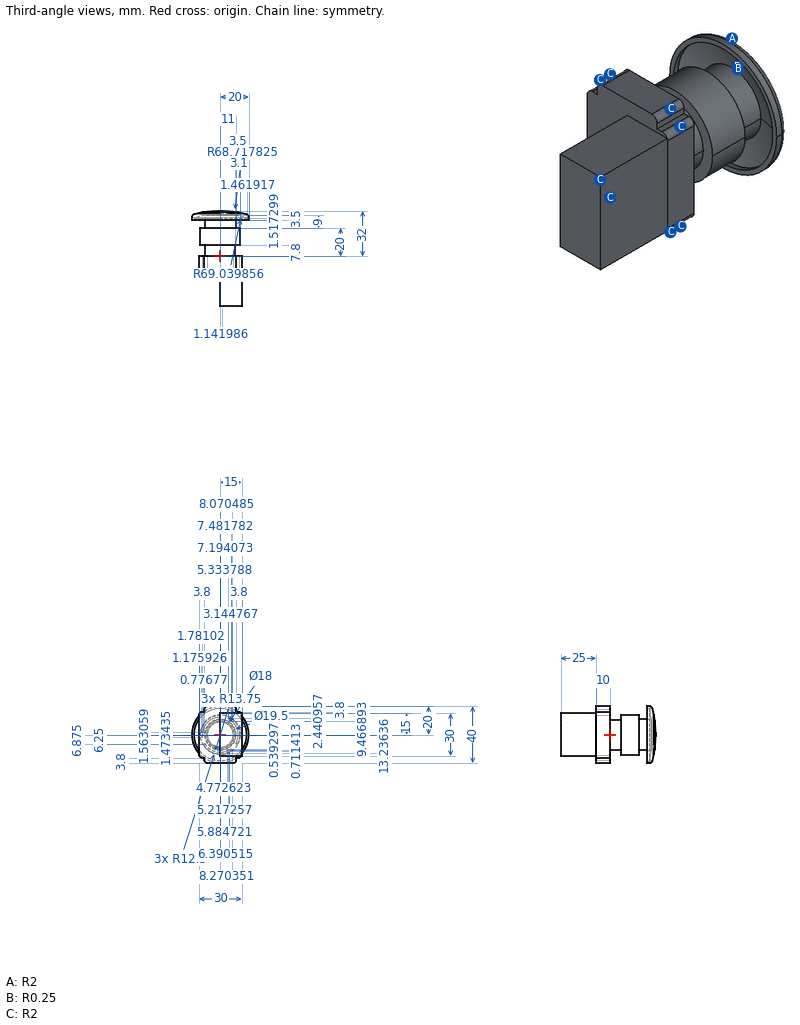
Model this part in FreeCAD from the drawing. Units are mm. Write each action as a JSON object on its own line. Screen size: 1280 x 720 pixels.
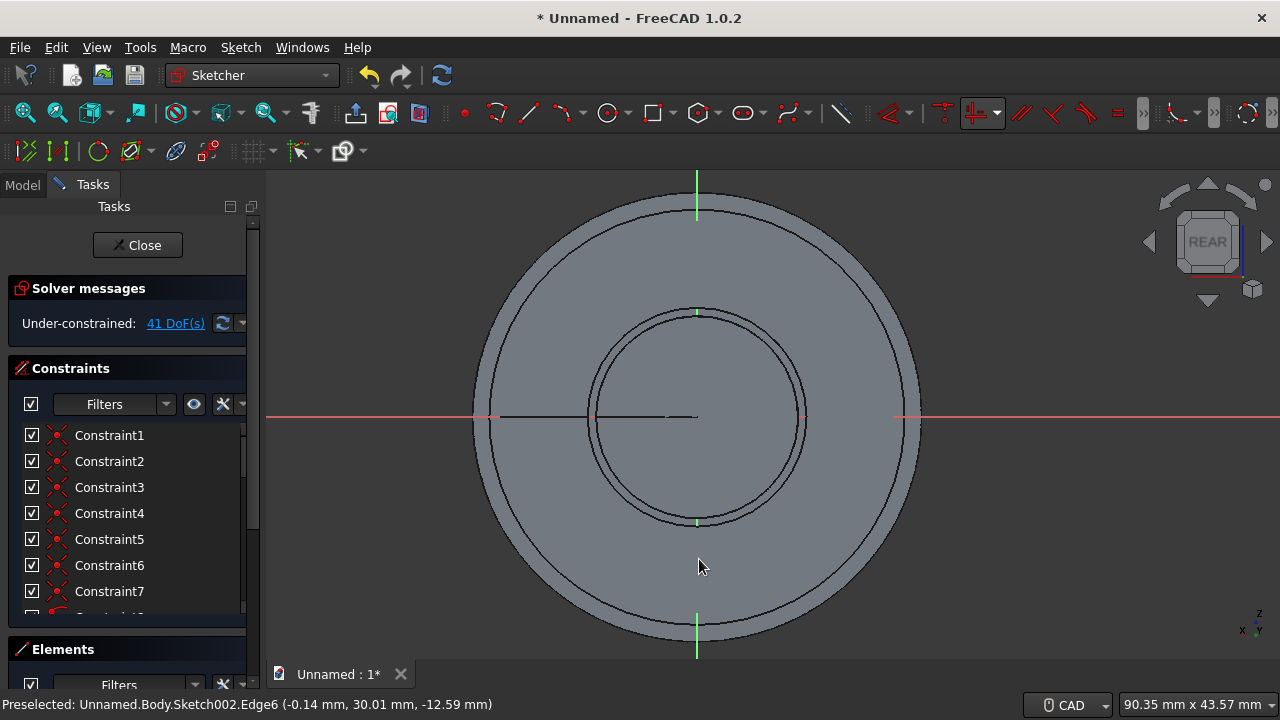
{"action": "left_click", "coordinate": [816, 344]}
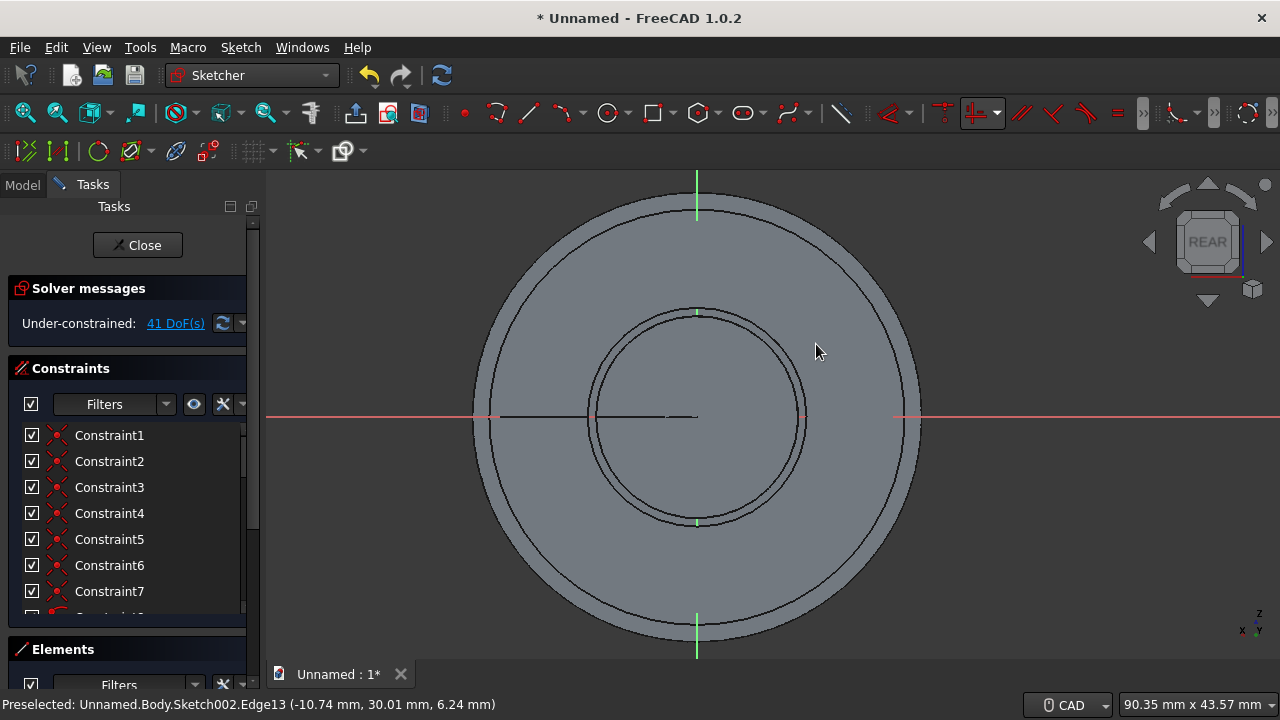
{"action": "left_click", "coordinate": [944, 114]}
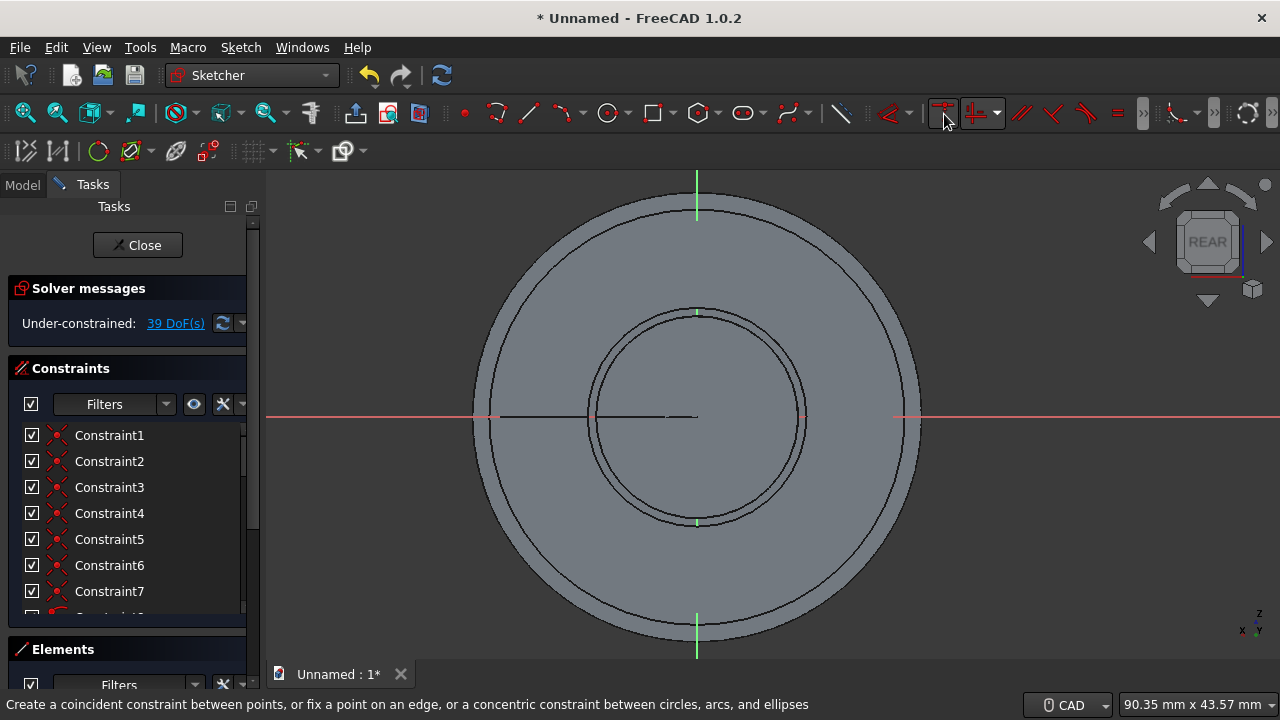
{"action": "left_click", "coordinate": [699, 558]}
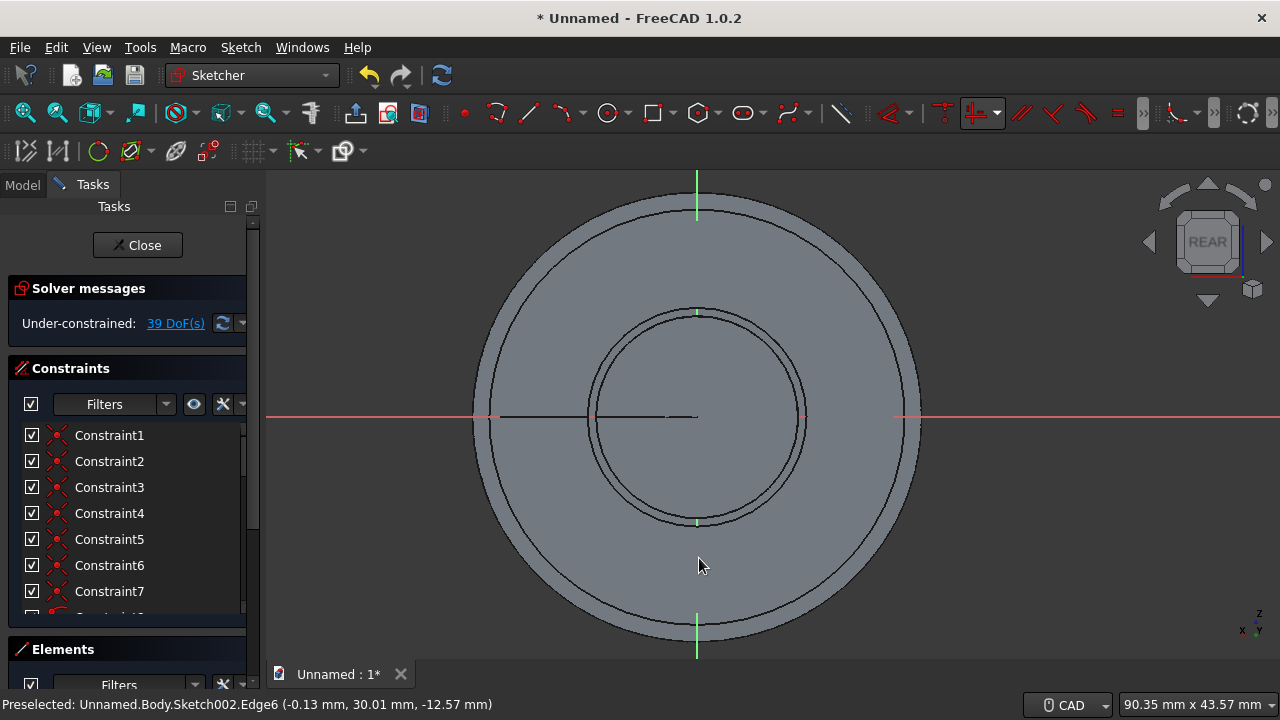
{"action": "left_click", "coordinate": [829, 337]}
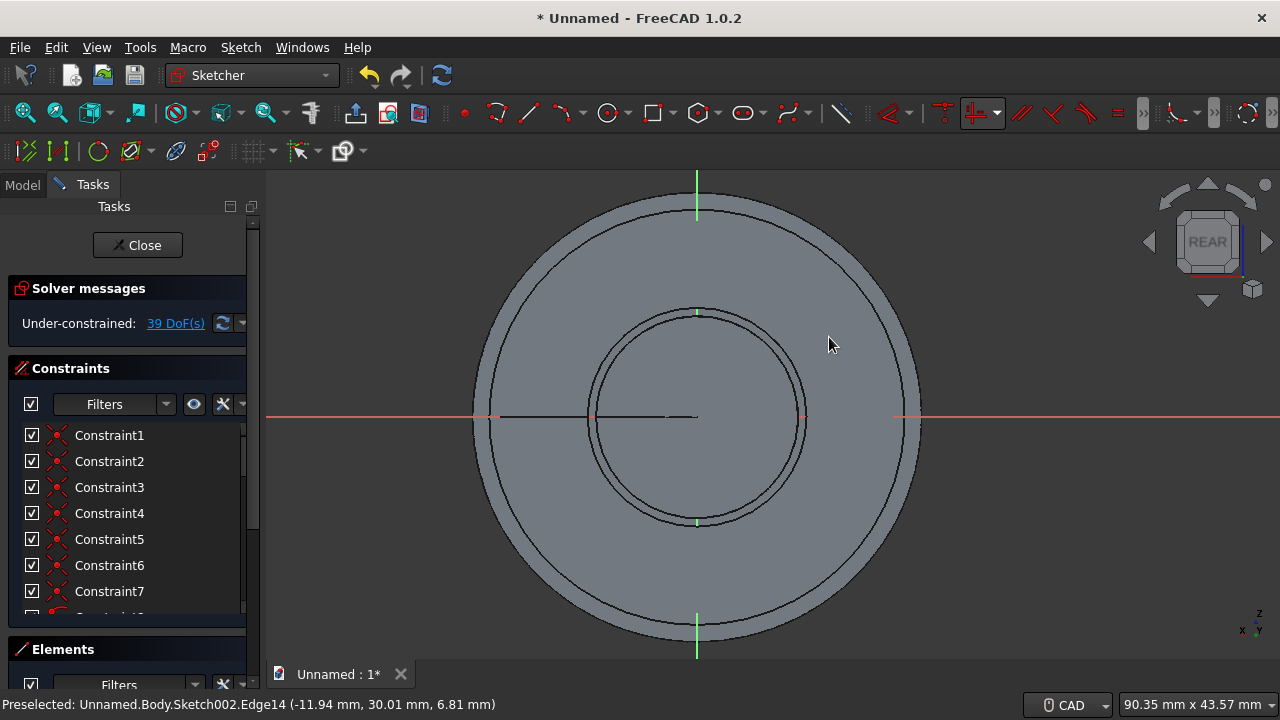
{"action": "left_click", "coordinate": [944, 114]}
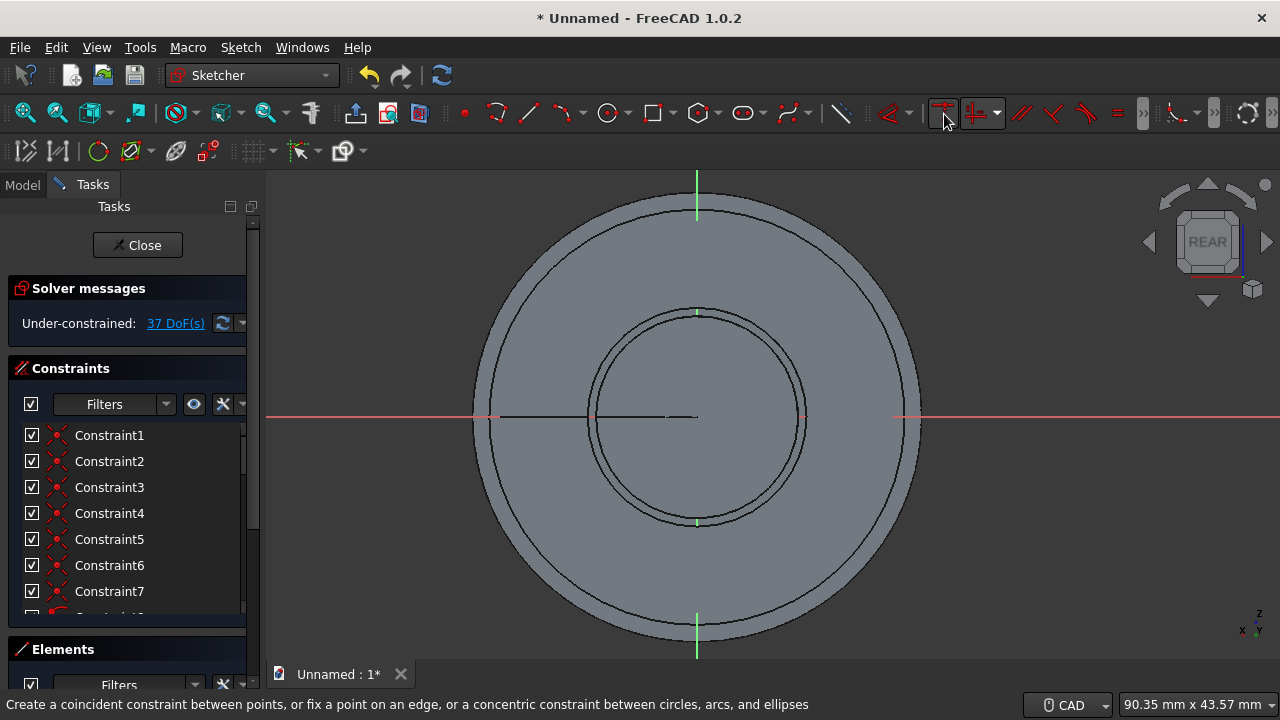
{"action": "left_click", "coordinate": [699, 558]}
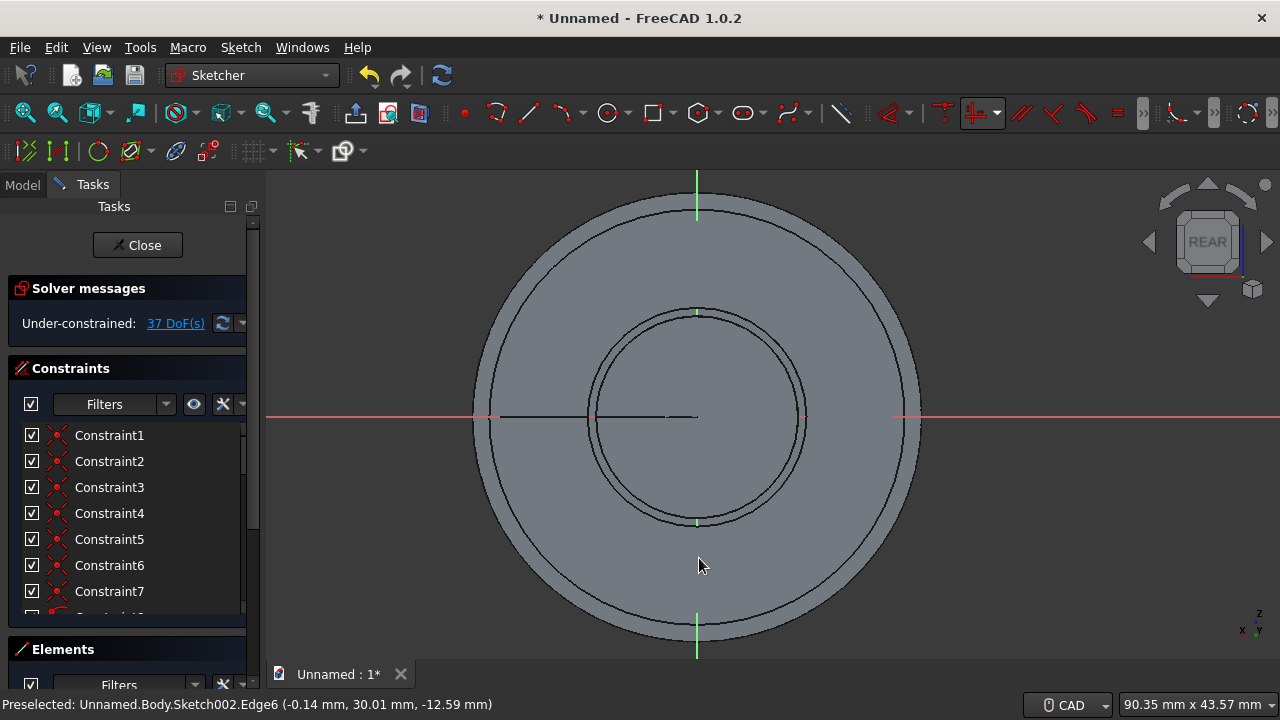
{"action": "left_click", "coordinate": [574, 352]}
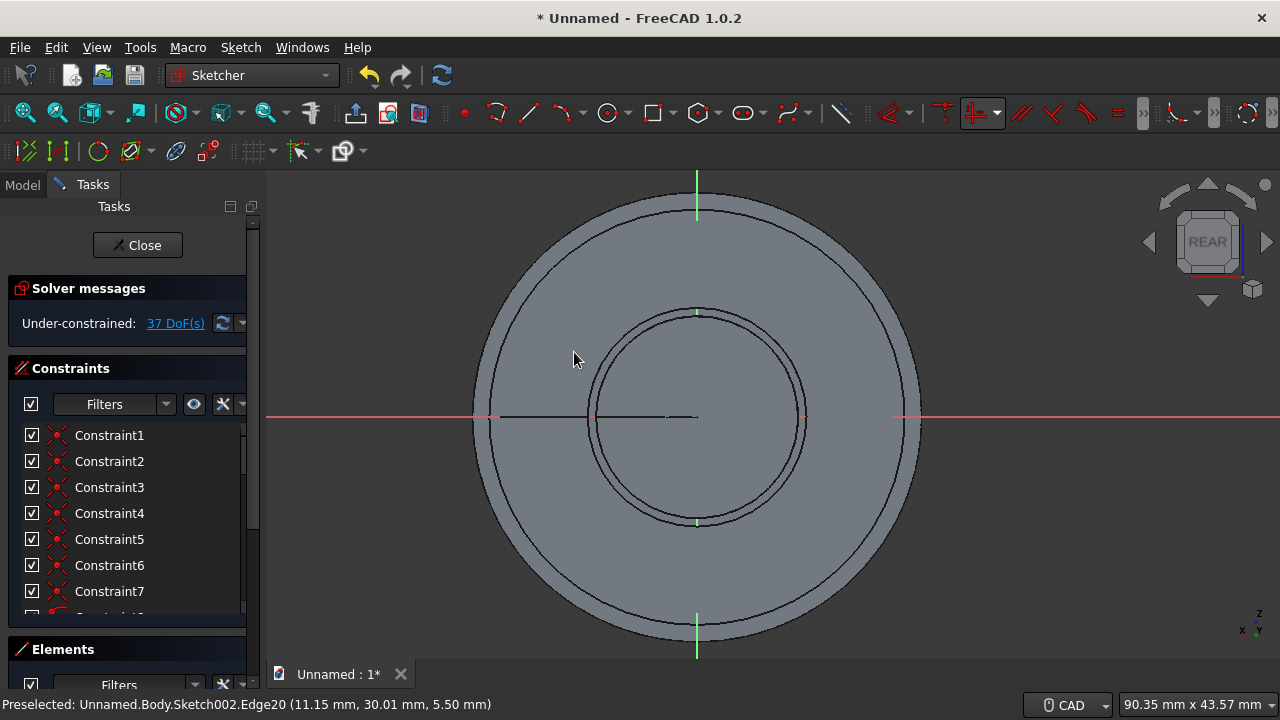
{"action": "left_click", "coordinate": [944, 114]}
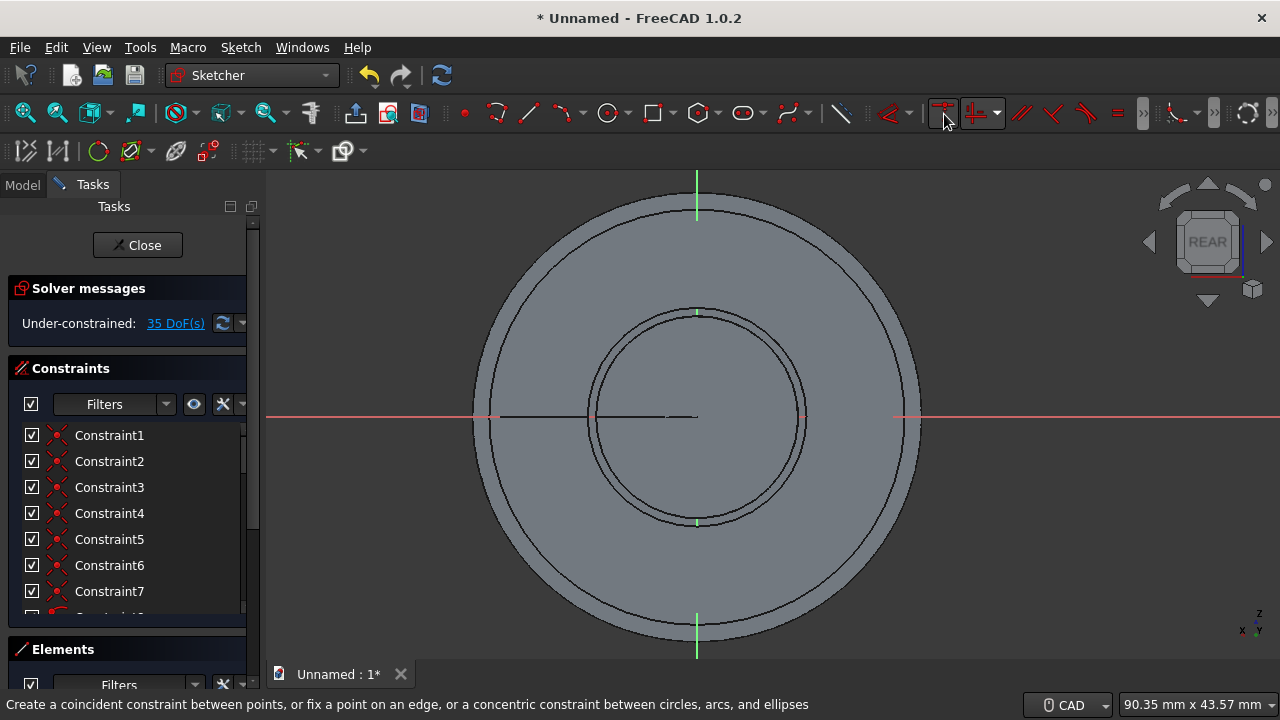
{"action": "left_click", "coordinate": [699, 558]}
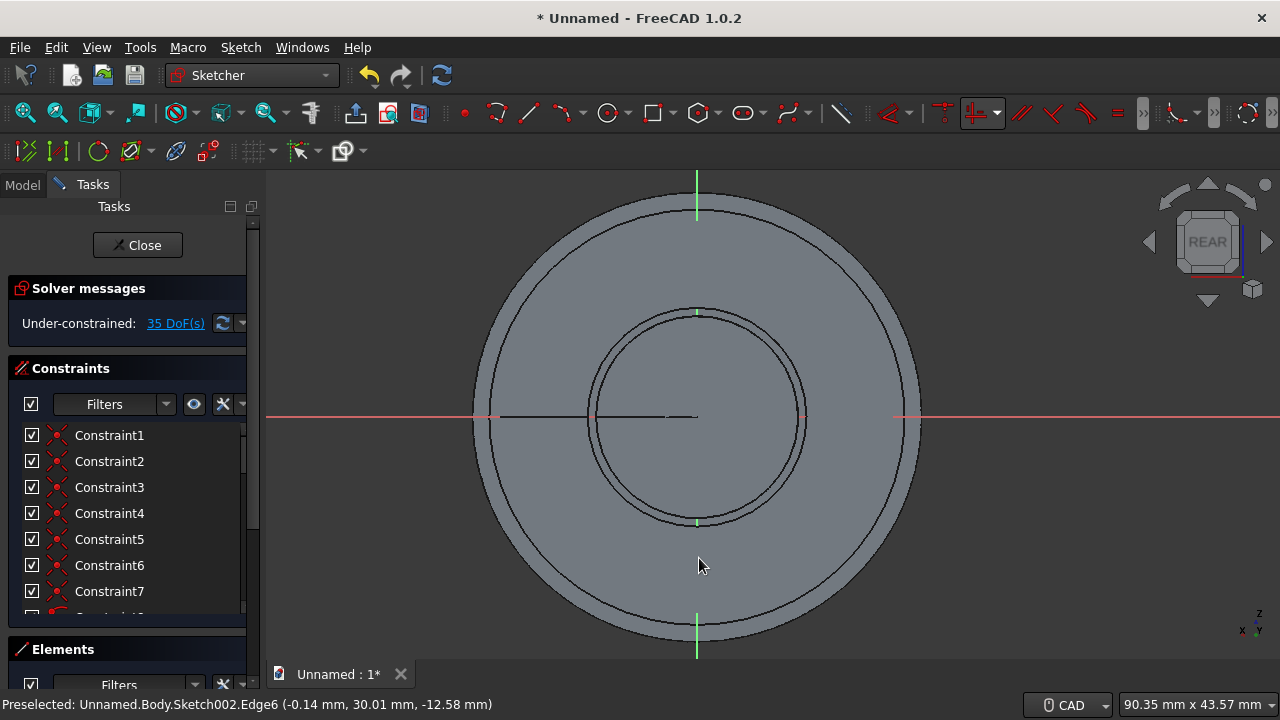
{"action": "left_click", "coordinate": [562, 343]}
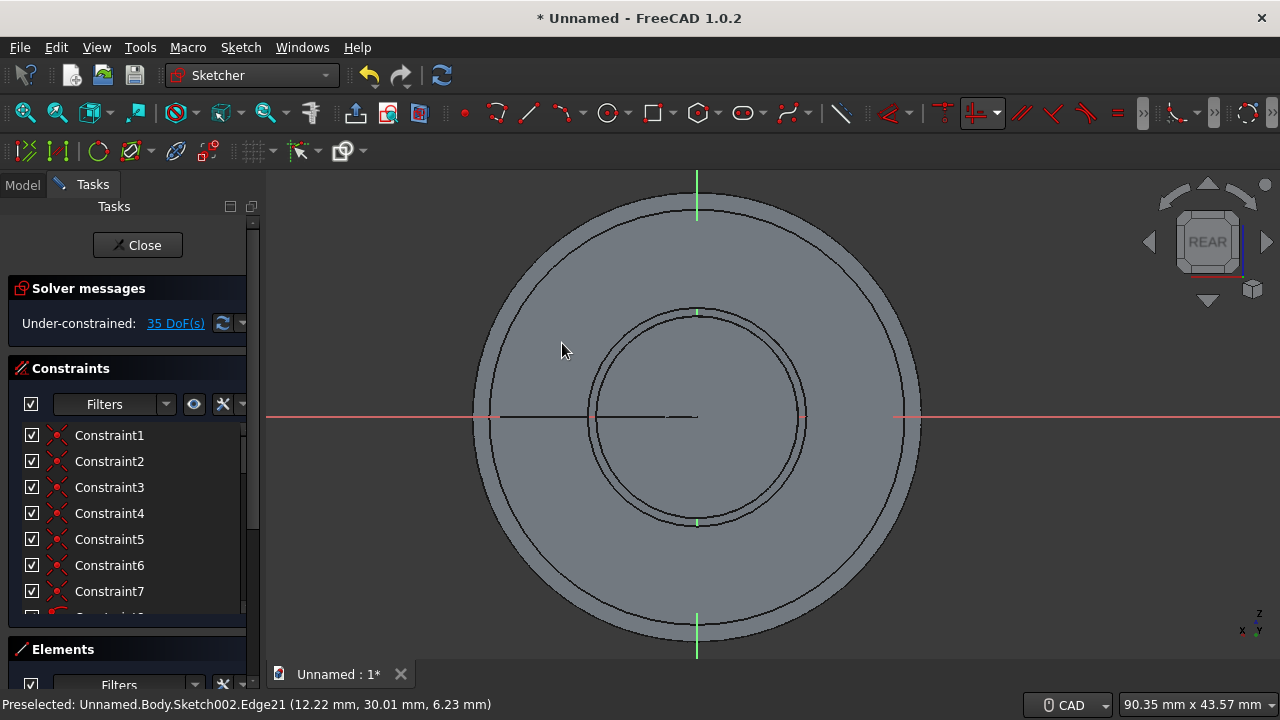
{"action": "left_click", "coordinate": [944, 114]}